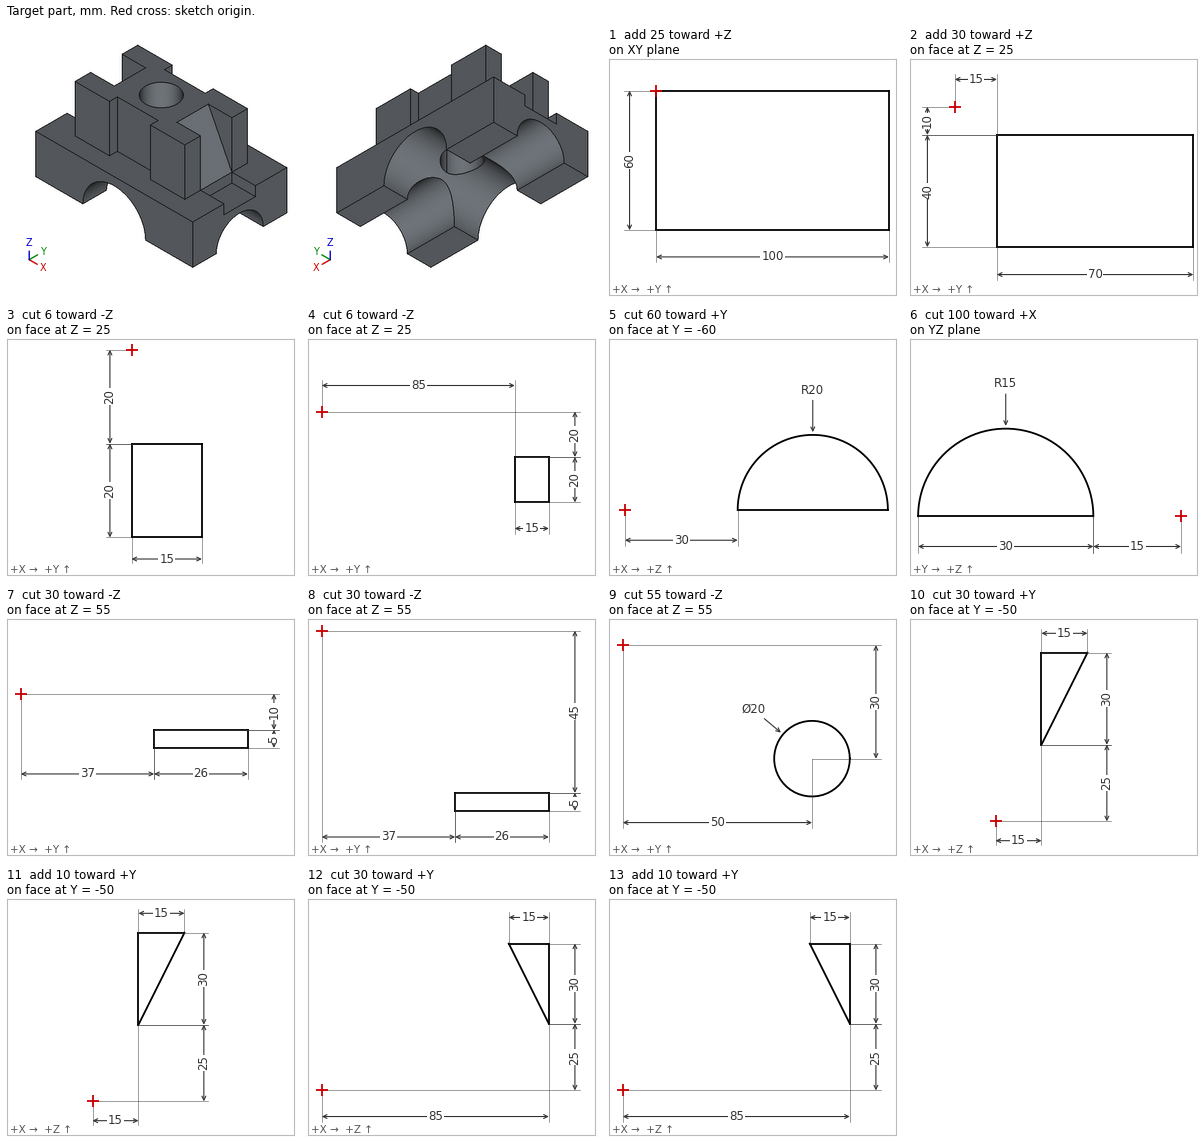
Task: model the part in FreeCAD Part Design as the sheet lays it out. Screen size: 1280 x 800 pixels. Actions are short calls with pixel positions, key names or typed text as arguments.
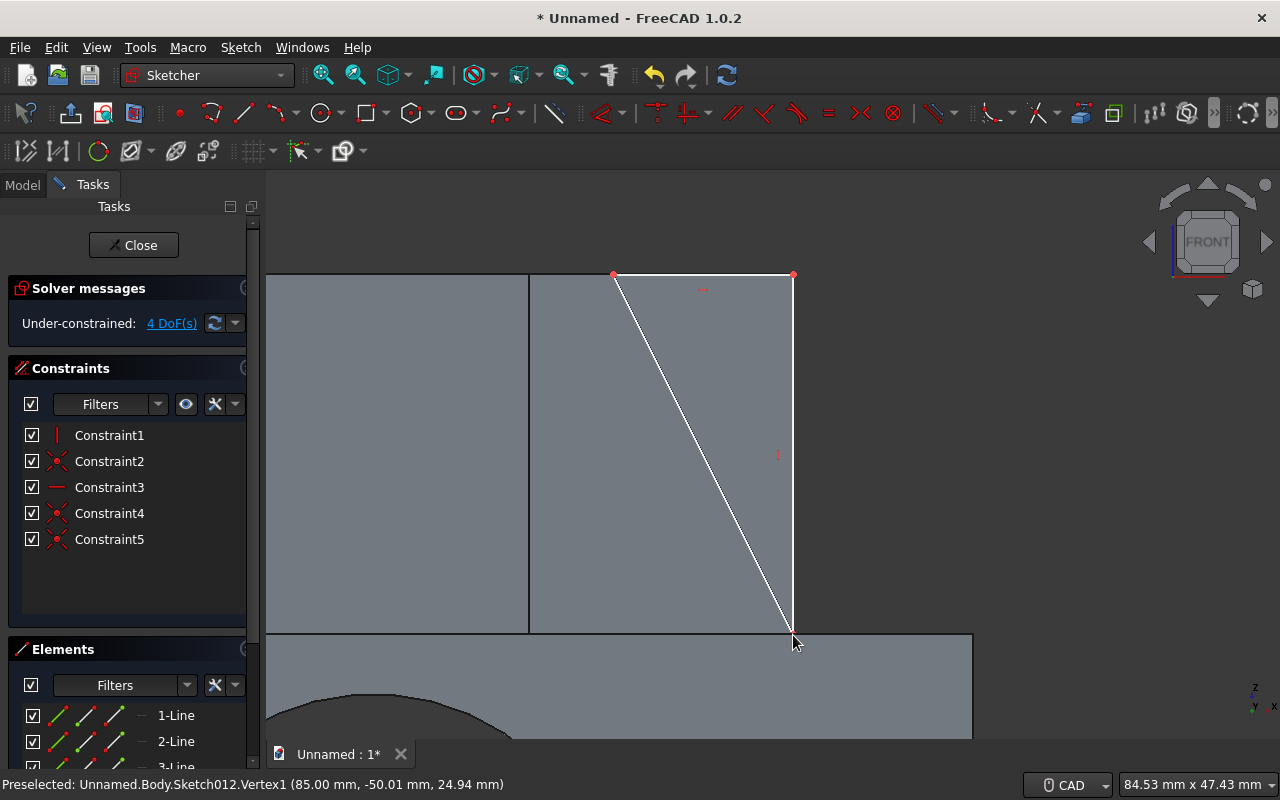
key(d)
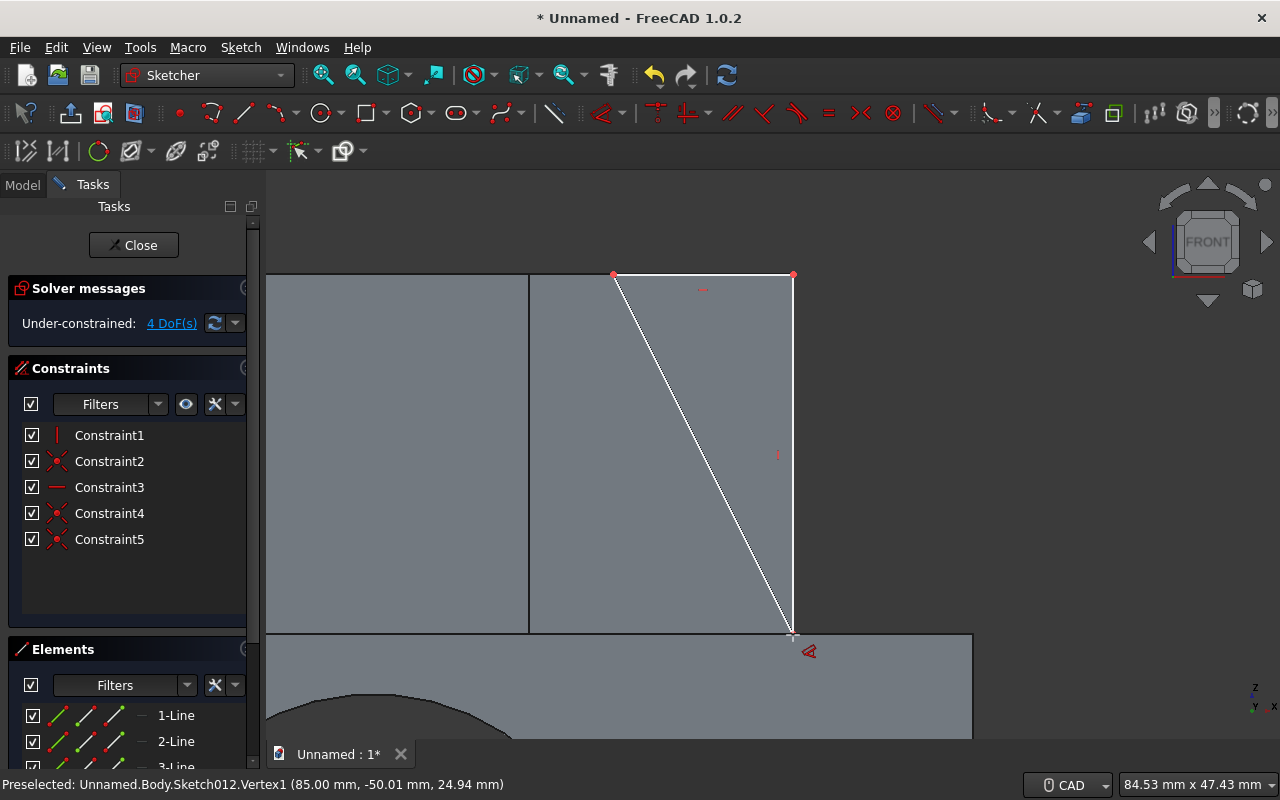
click(793, 527)
click(827, 455)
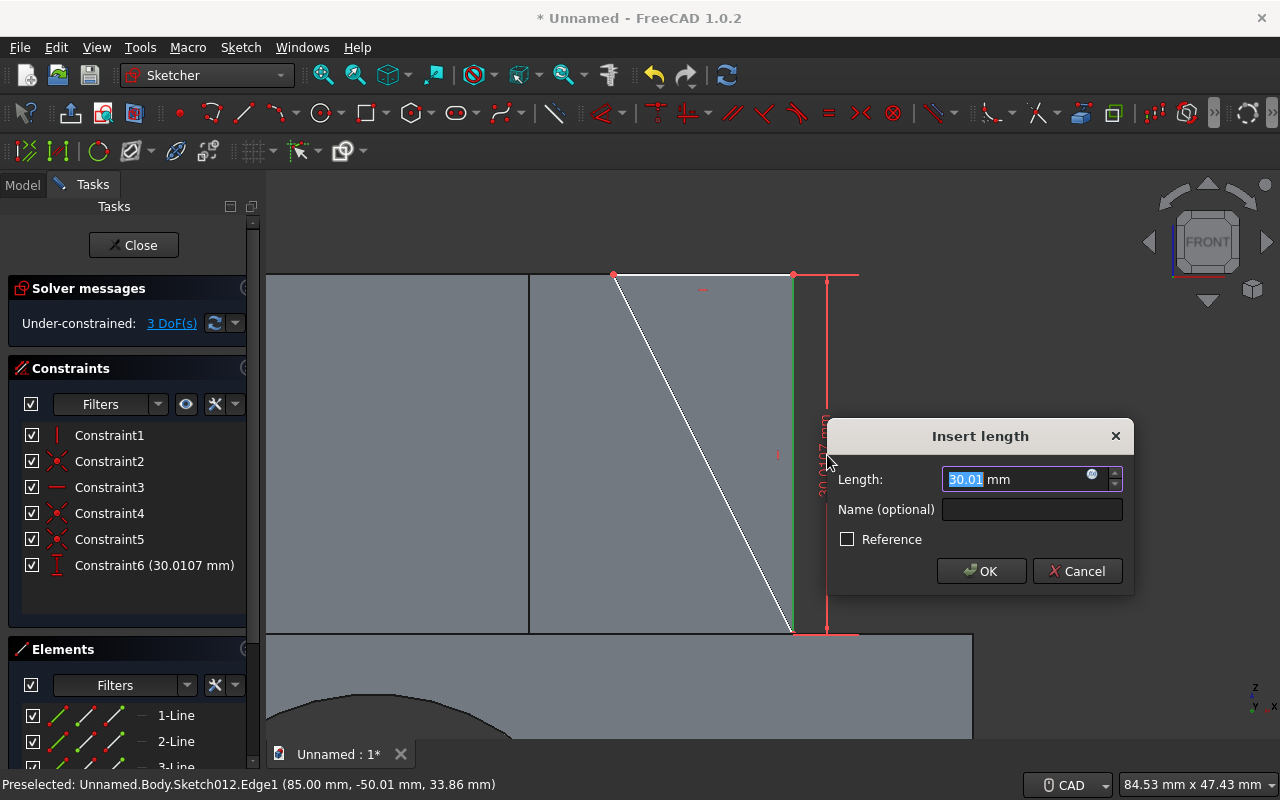
text(30)
key(Return)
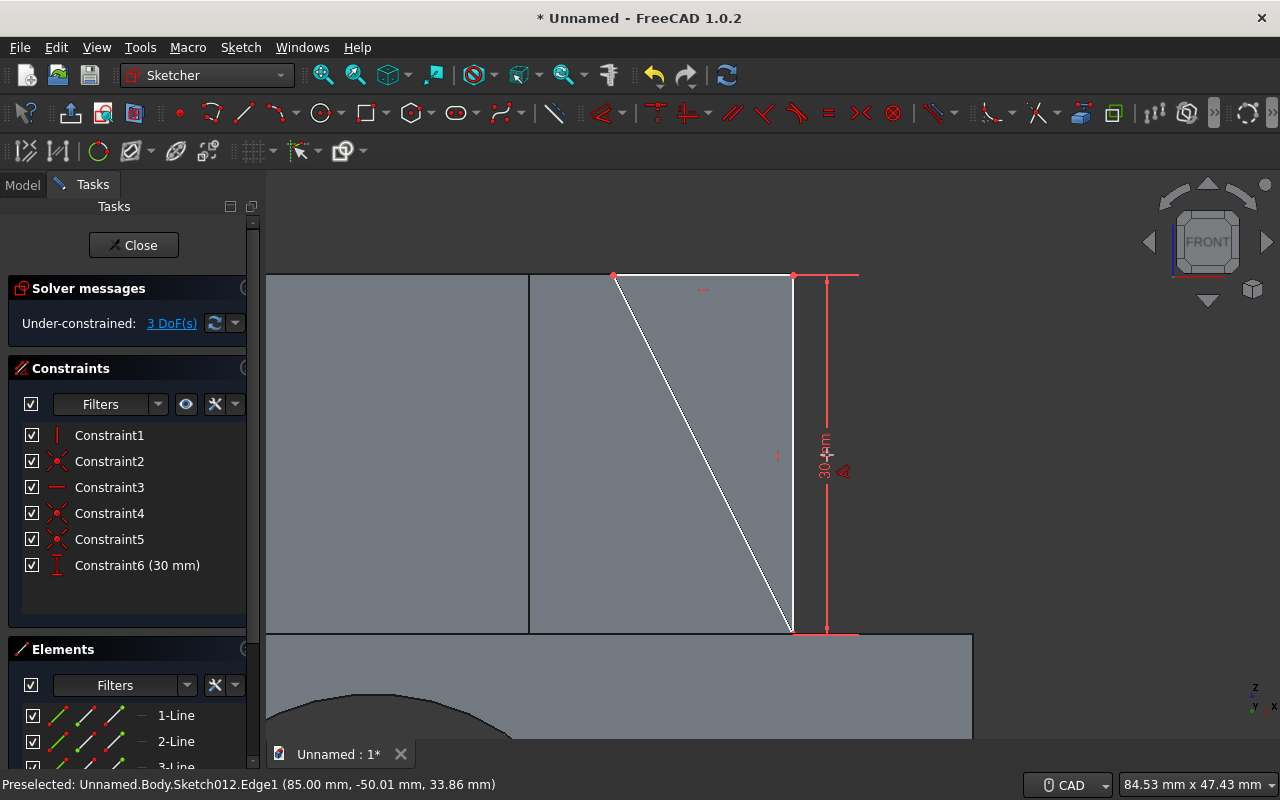
click(739, 275)
click(703, 241)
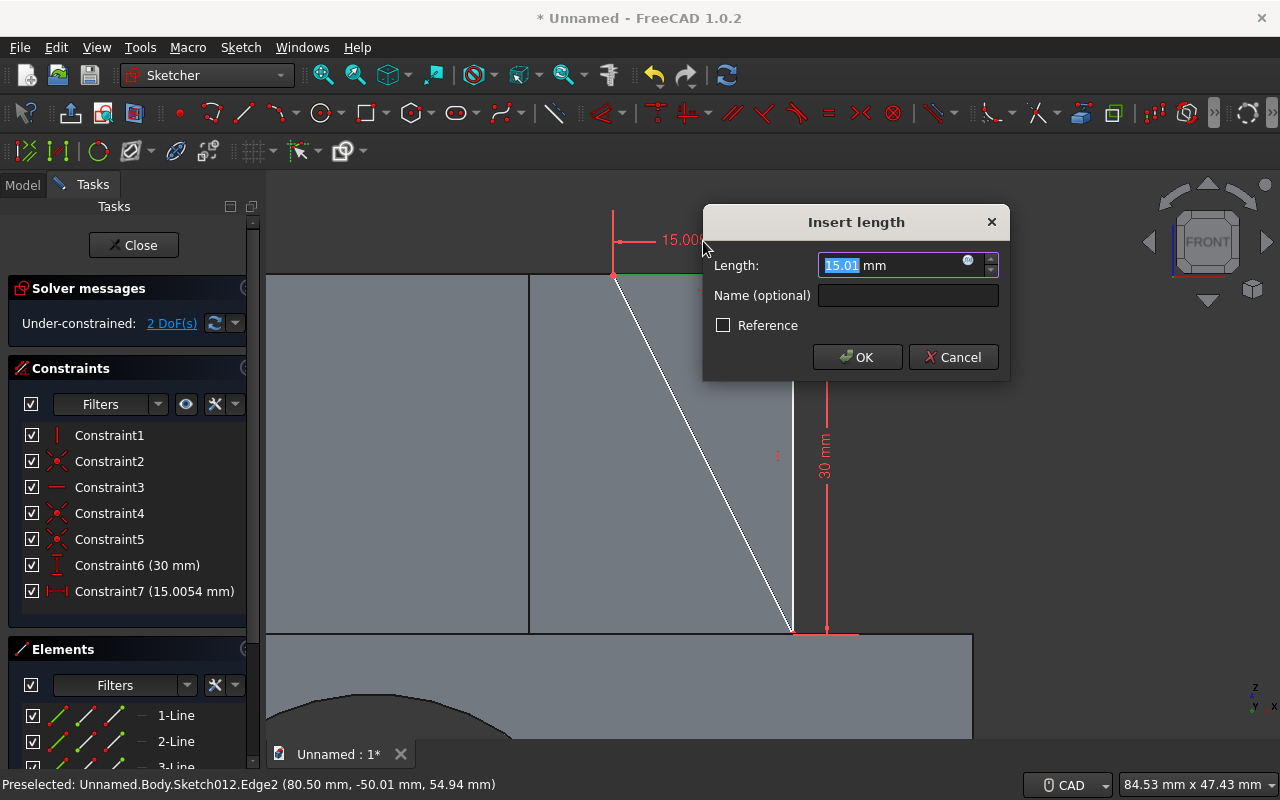
text(15)
key(Return)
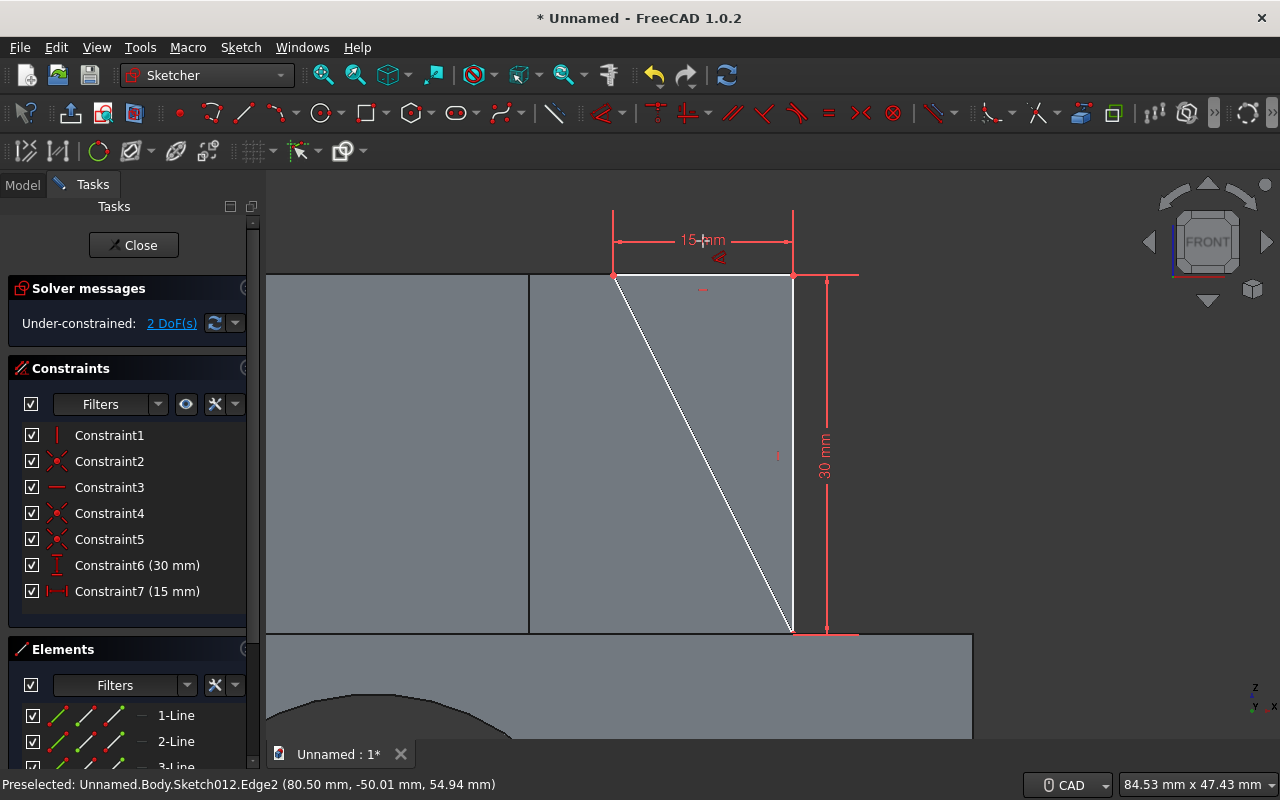
click(793, 635)
click(544, 601)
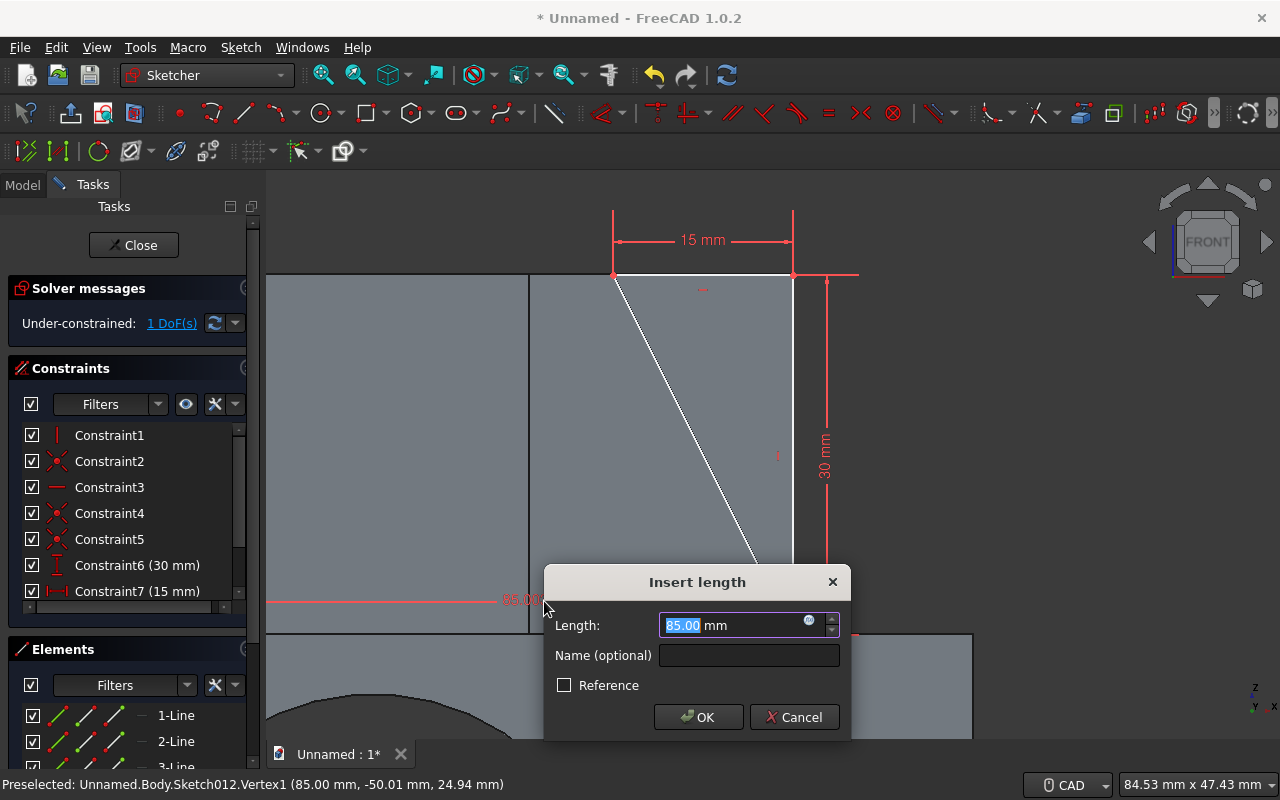
text(85)
key(Return)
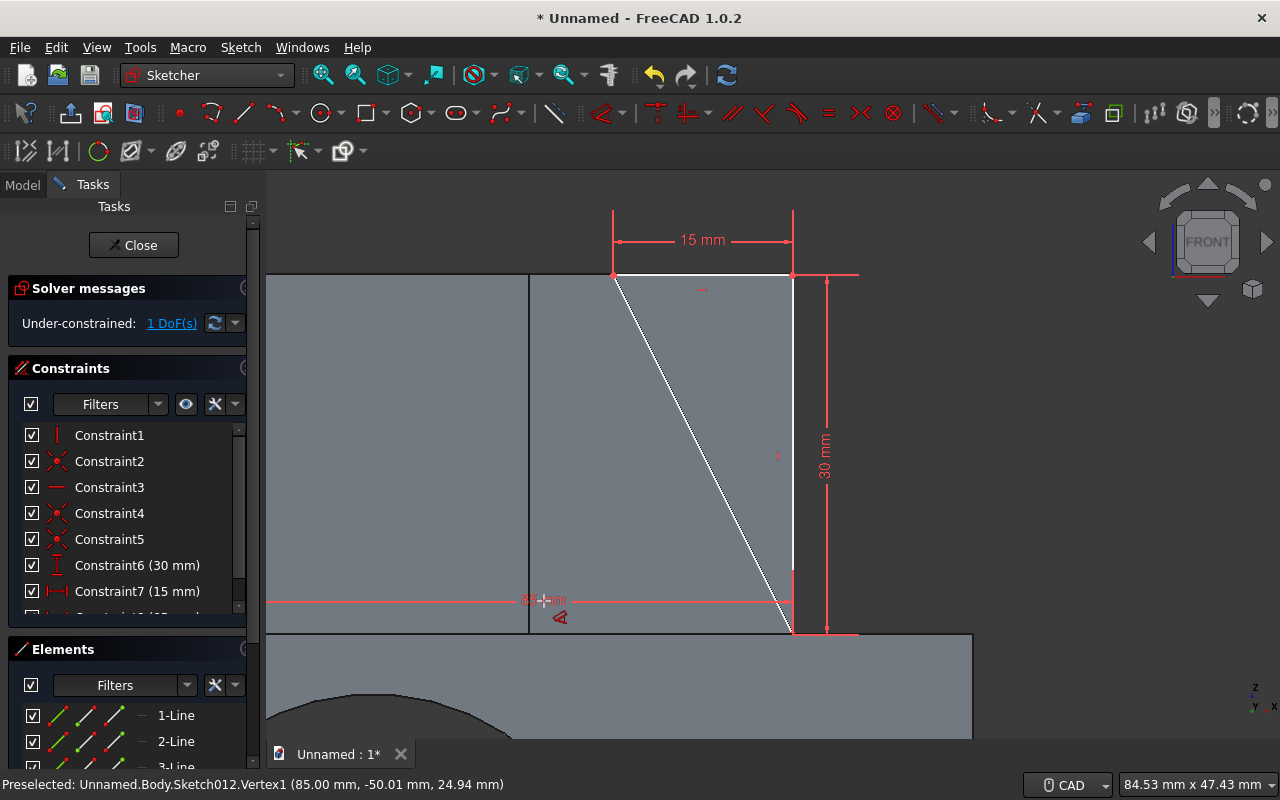
click(793, 635)
click(827, 673)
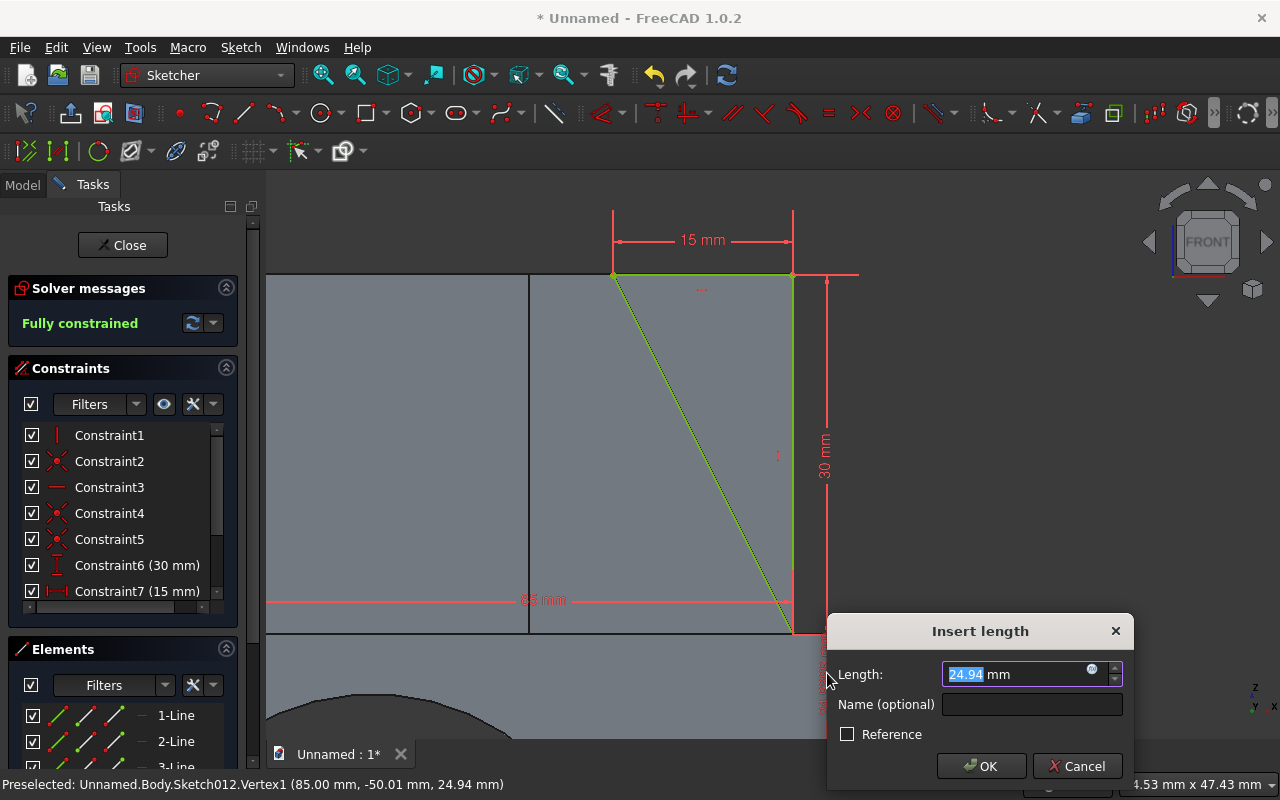
text(25)
key(Return)
key(Escape)